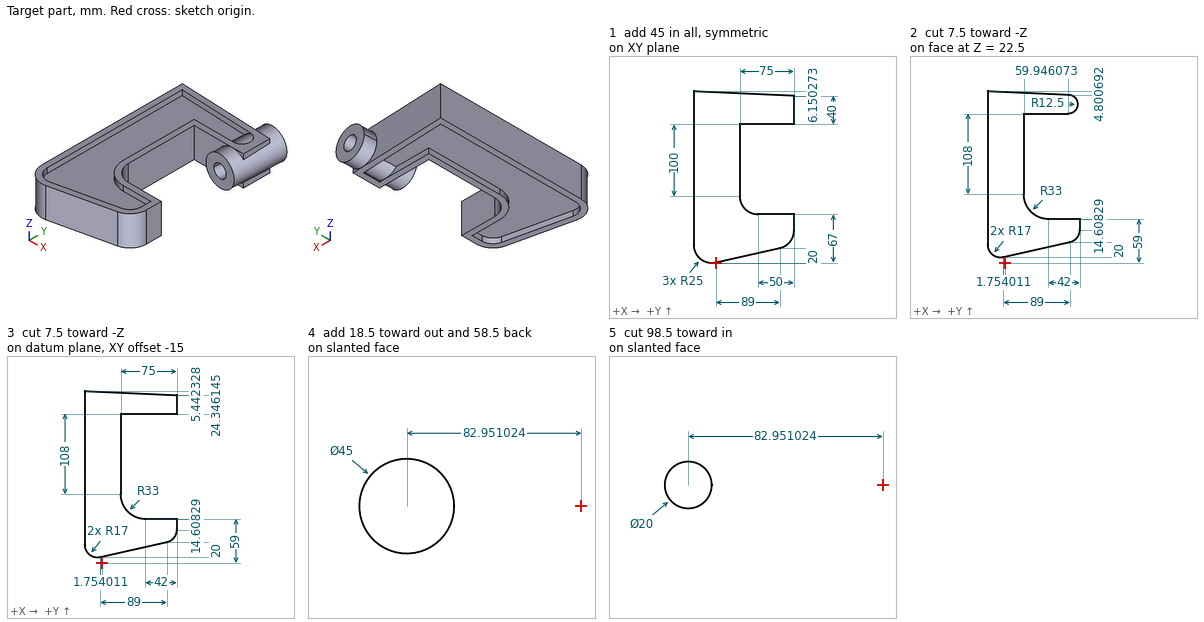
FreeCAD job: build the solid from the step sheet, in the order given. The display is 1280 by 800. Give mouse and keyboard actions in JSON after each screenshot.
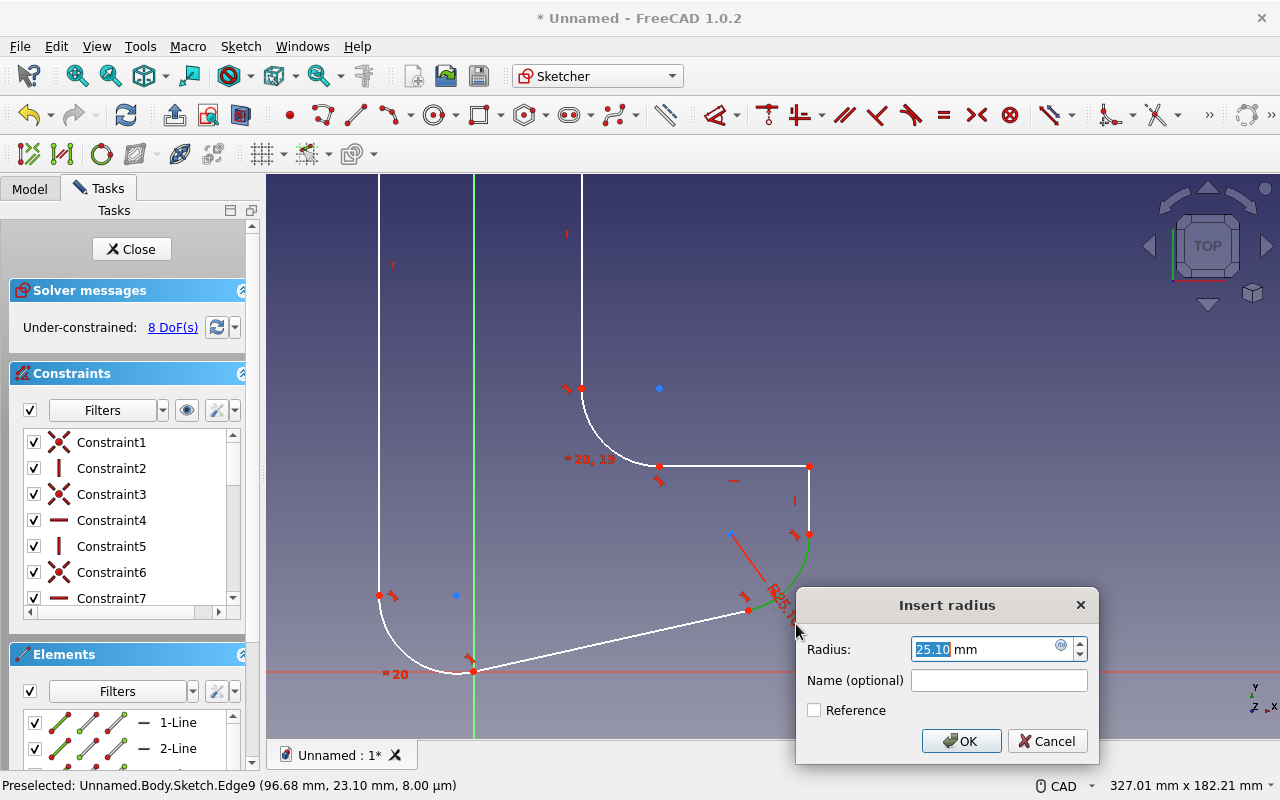
{"action": "type", "text": "25"}
{"action": "key", "text": "Return"}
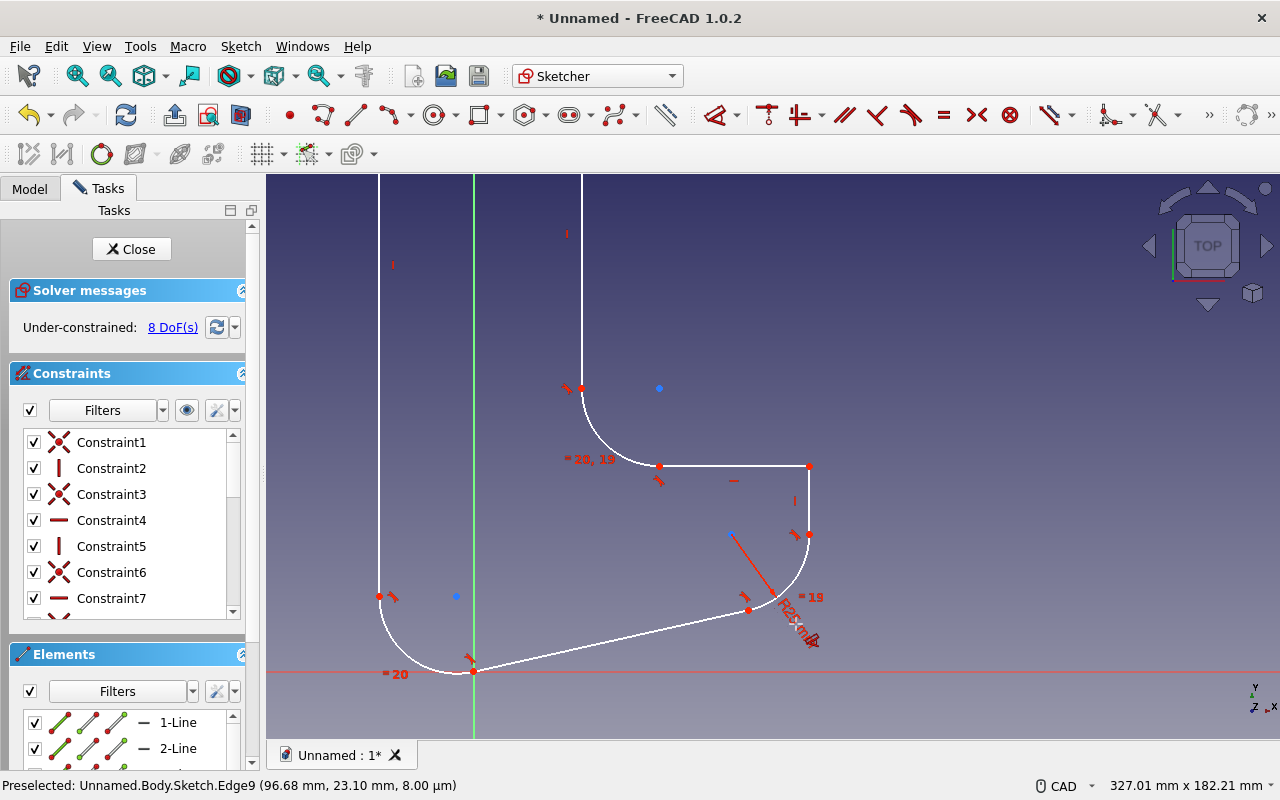
{"action": "left_click", "coordinate": [764, 466]}
{"action": "left_click", "coordinate": [734, 500]}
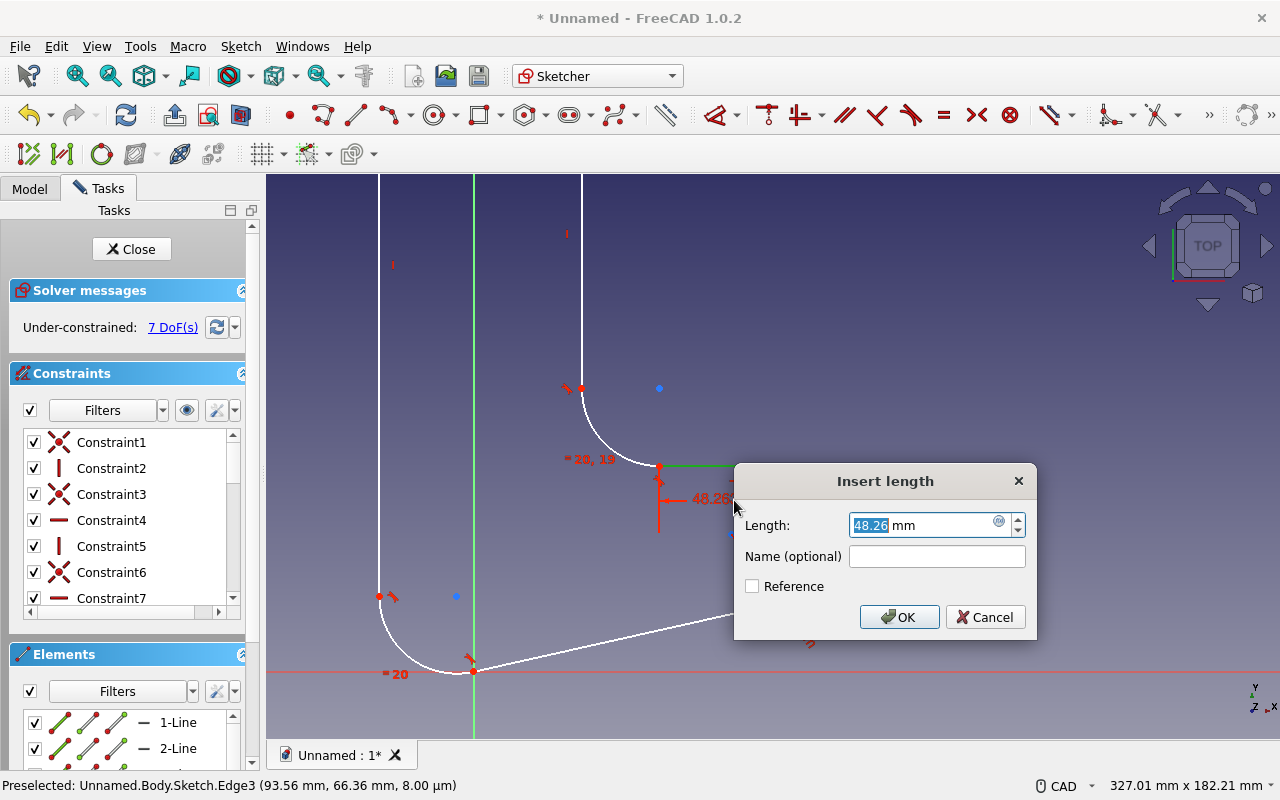
{"action": "type", "text": "50"}
{"action": "key", "text": "Return"}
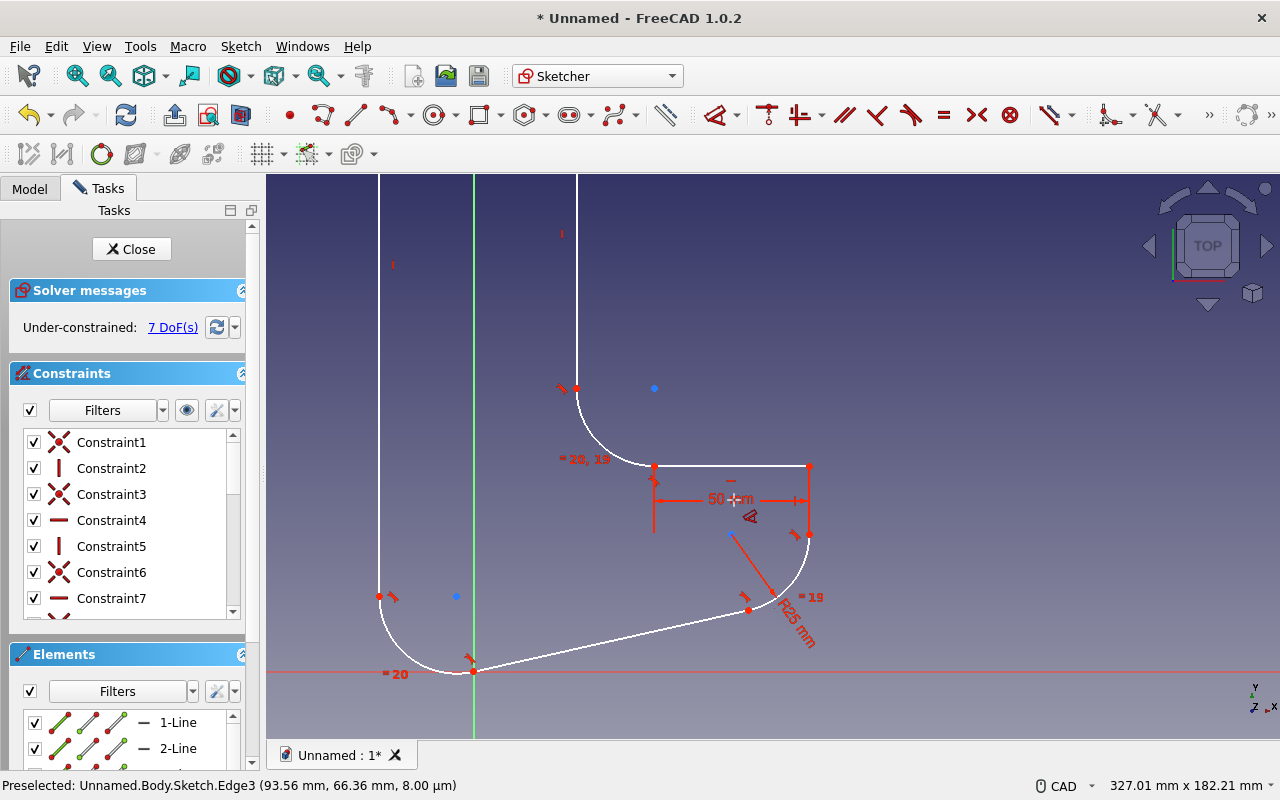
{"action": "scroll", "coordinate": [794, 582], "scroll_direction": "down", "scroll_amount": 4}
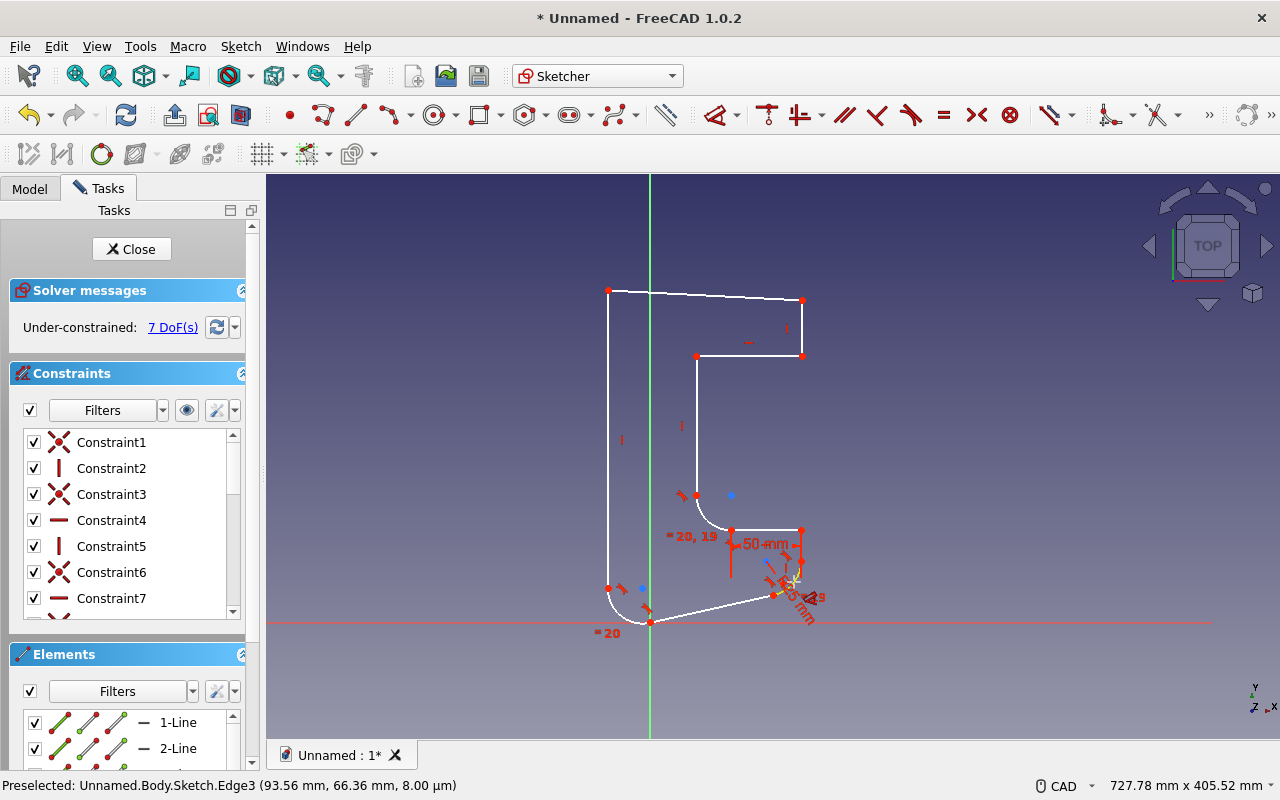
{"action": "left_click", "coordinate": [728, 356]}
{"action": "left_click", "coordinate": [749, 322]}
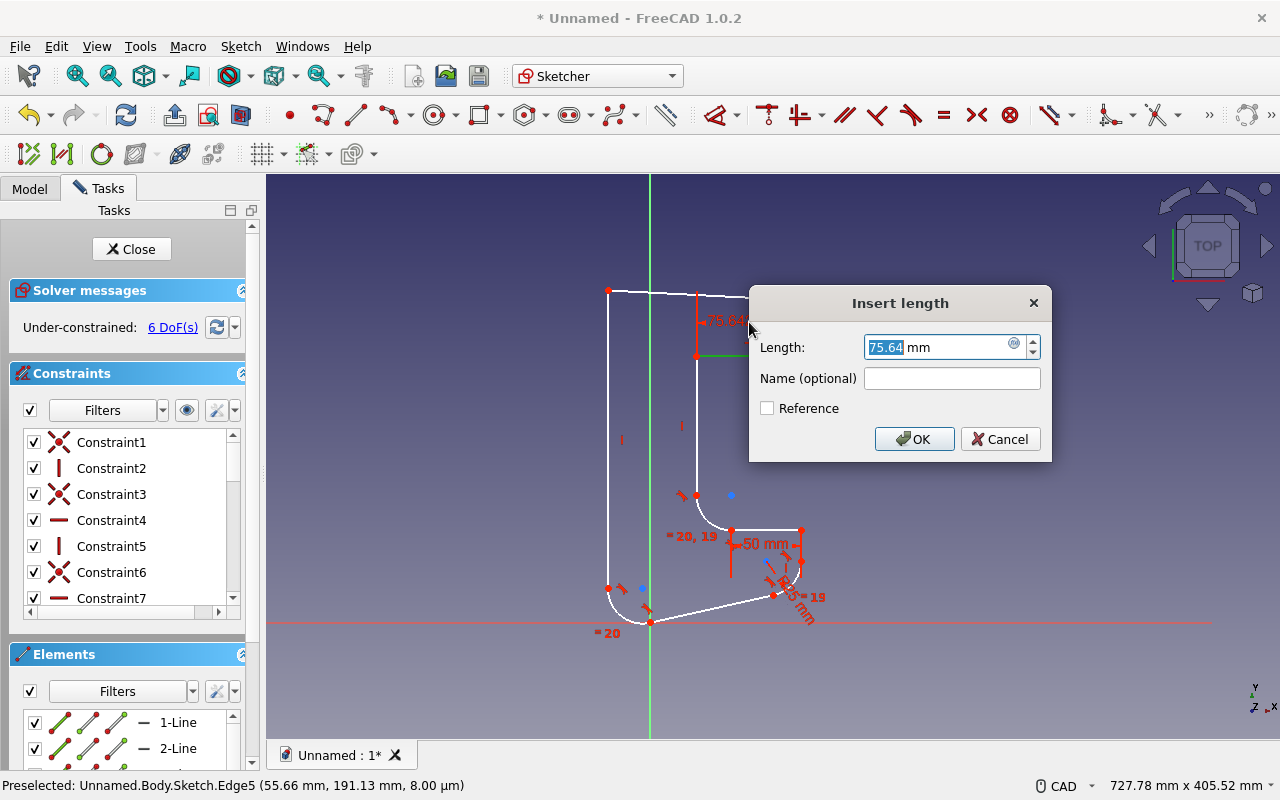
{"action": "type", "text": "75"}
{"action": "key", "text": "Return"}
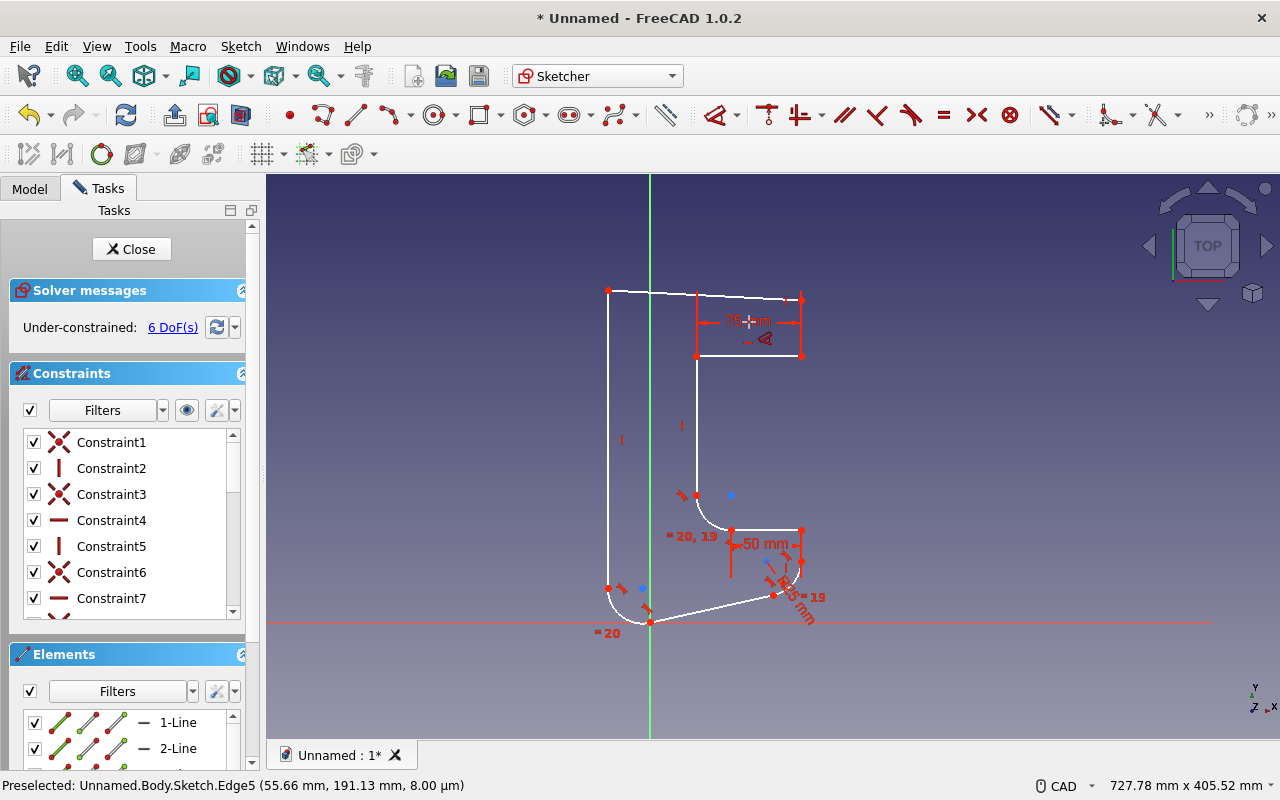
{"action": "left_click", "coordinate": [801, 340]}
{"action": "left_click", "coordinate": [835, 328]}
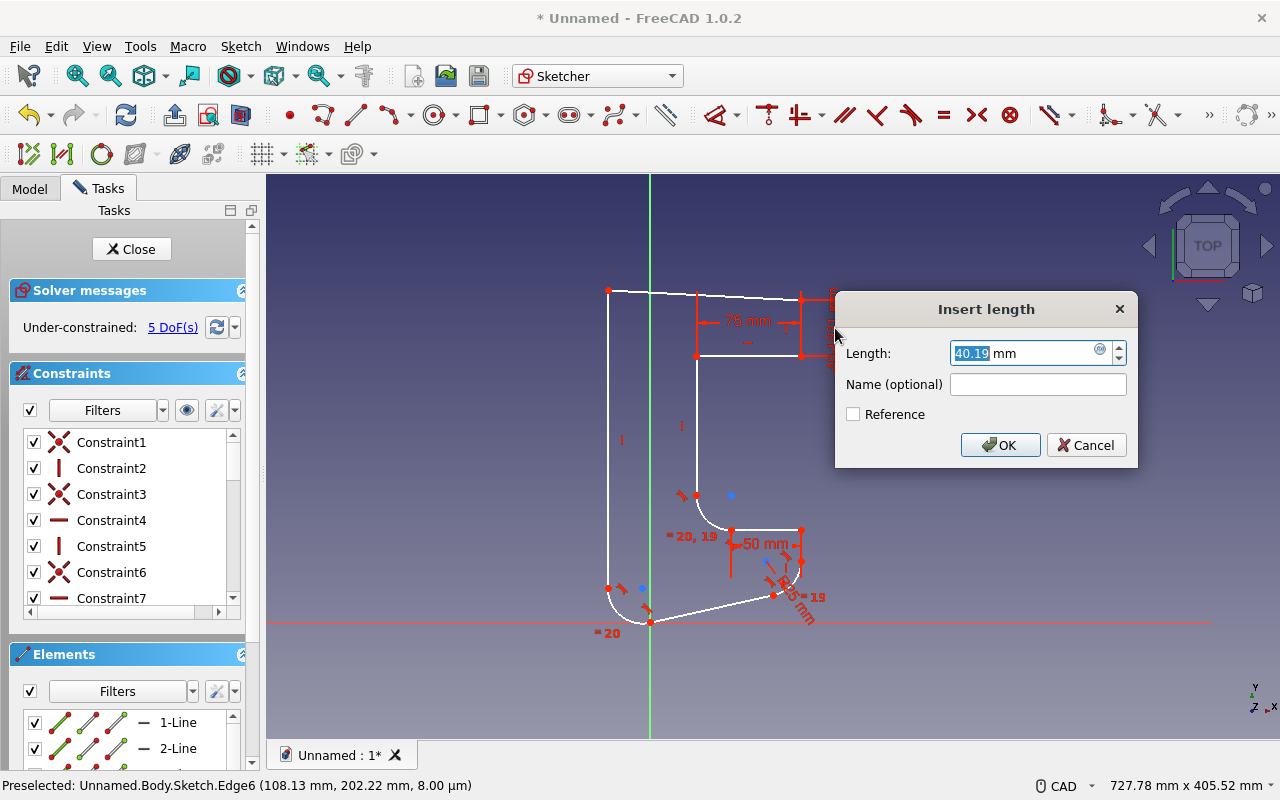
{"action": "type", "text": "40"}
{"action": "key", "text": "Return"}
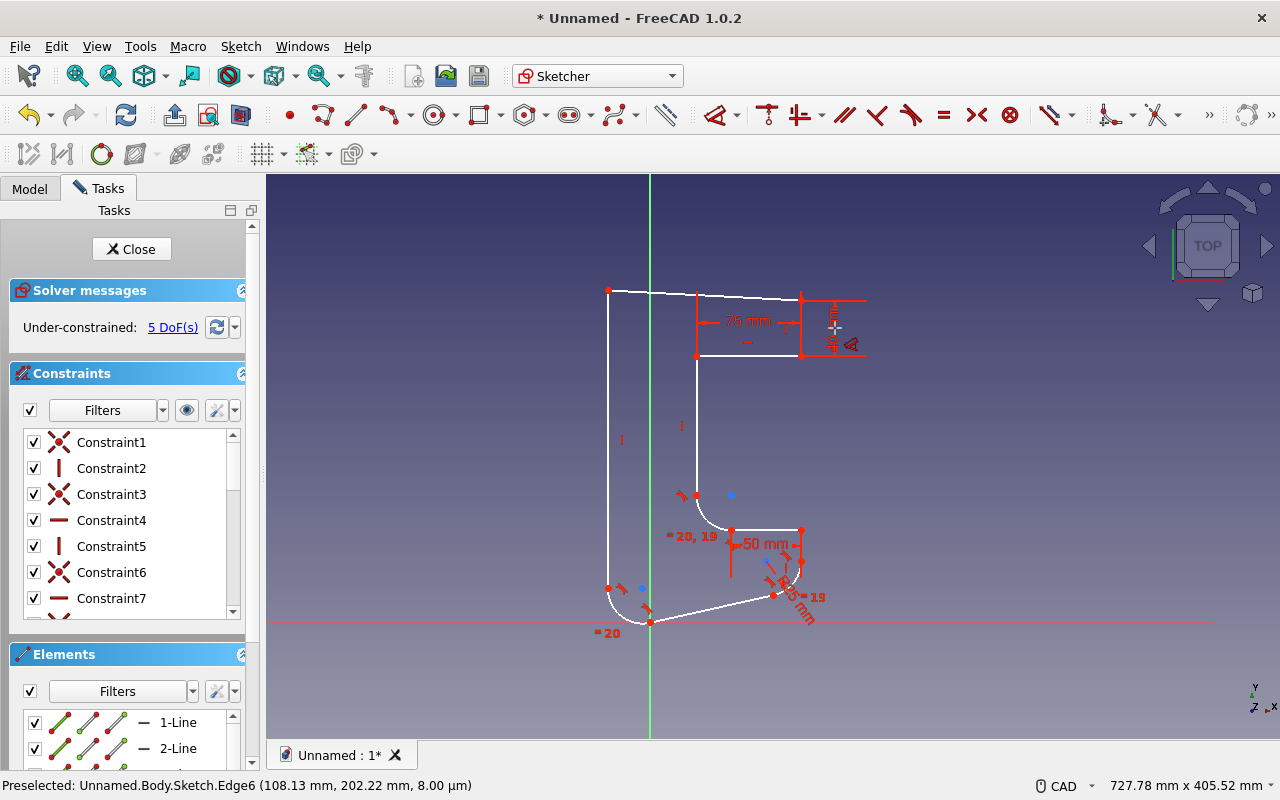
{"action": "left_click", "coordinate": [697, 454]}
{"action": "left_click", "coordinate": [731, 426]}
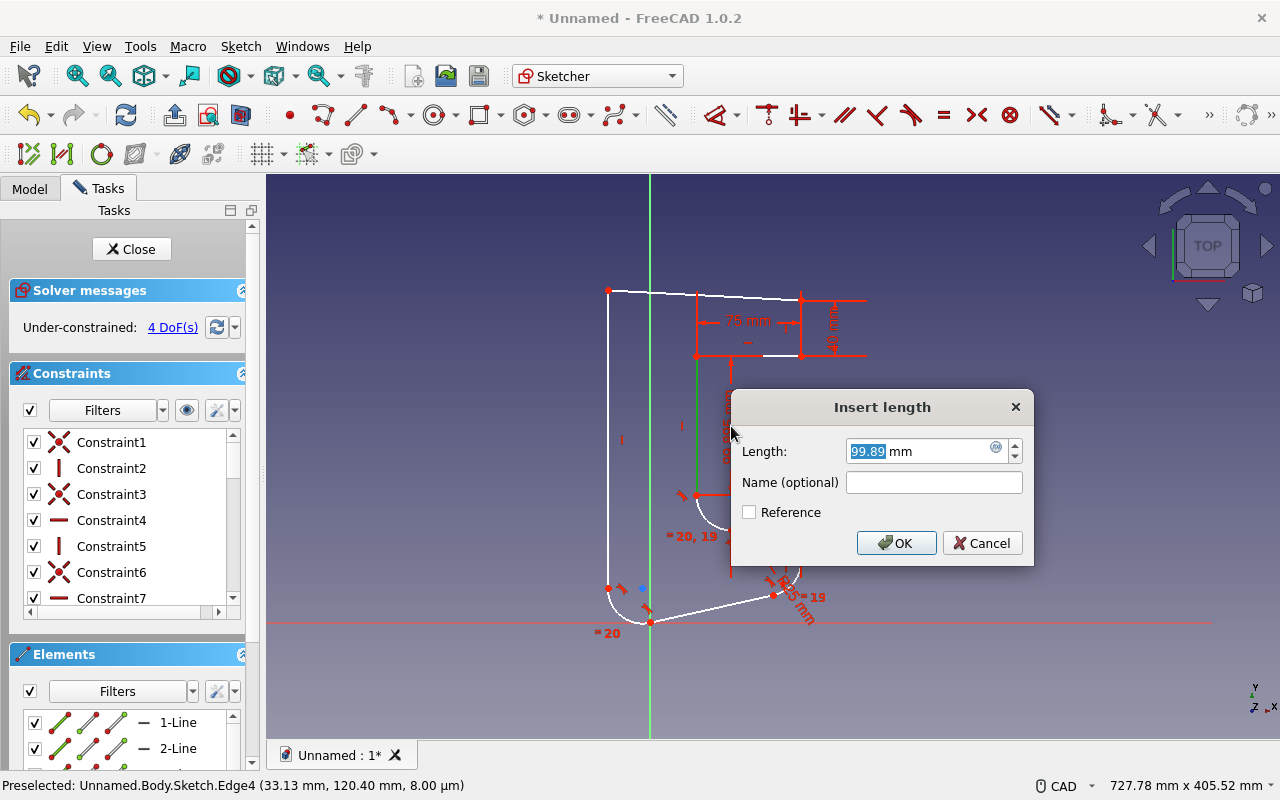
{"action": "type", "text": "100"}
{"action": "key", "text": "Return"}